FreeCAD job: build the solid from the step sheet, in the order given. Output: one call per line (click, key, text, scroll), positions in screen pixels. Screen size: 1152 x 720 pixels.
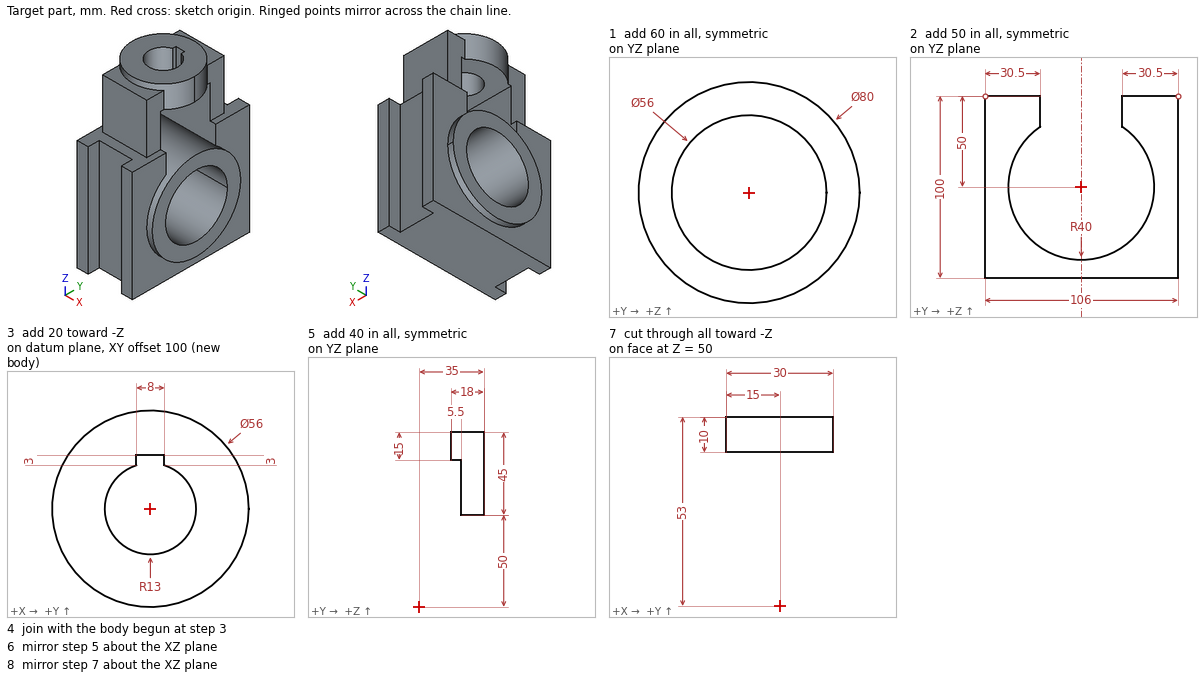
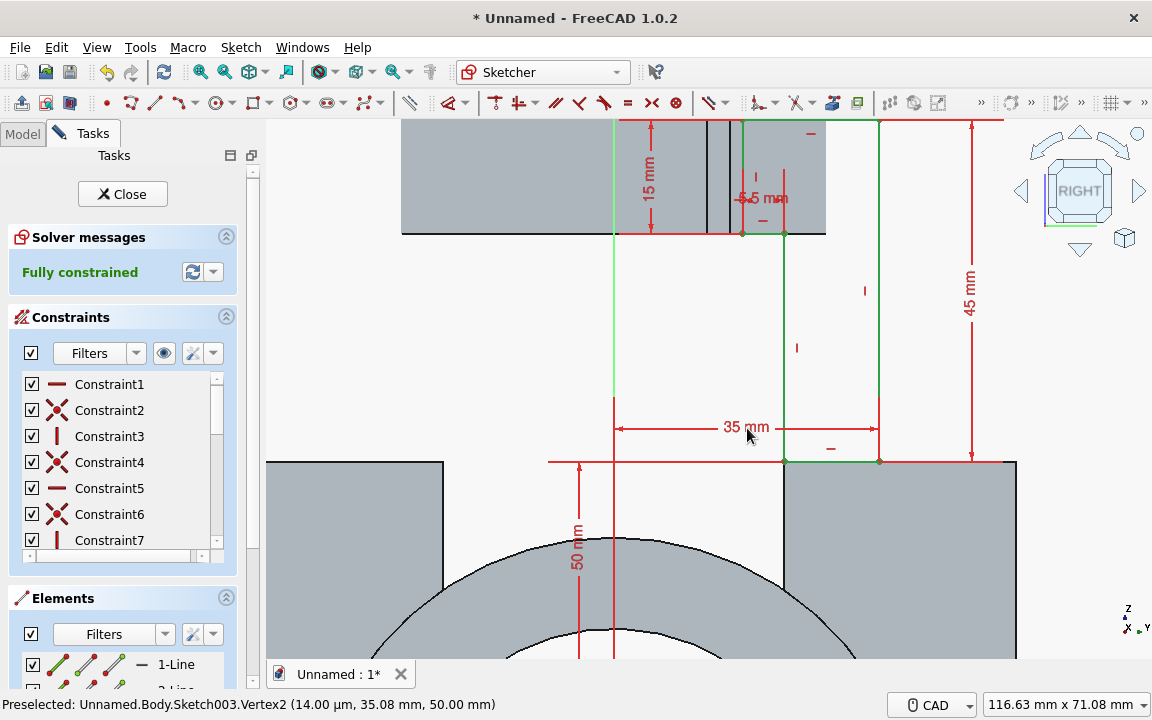
click(123, 194)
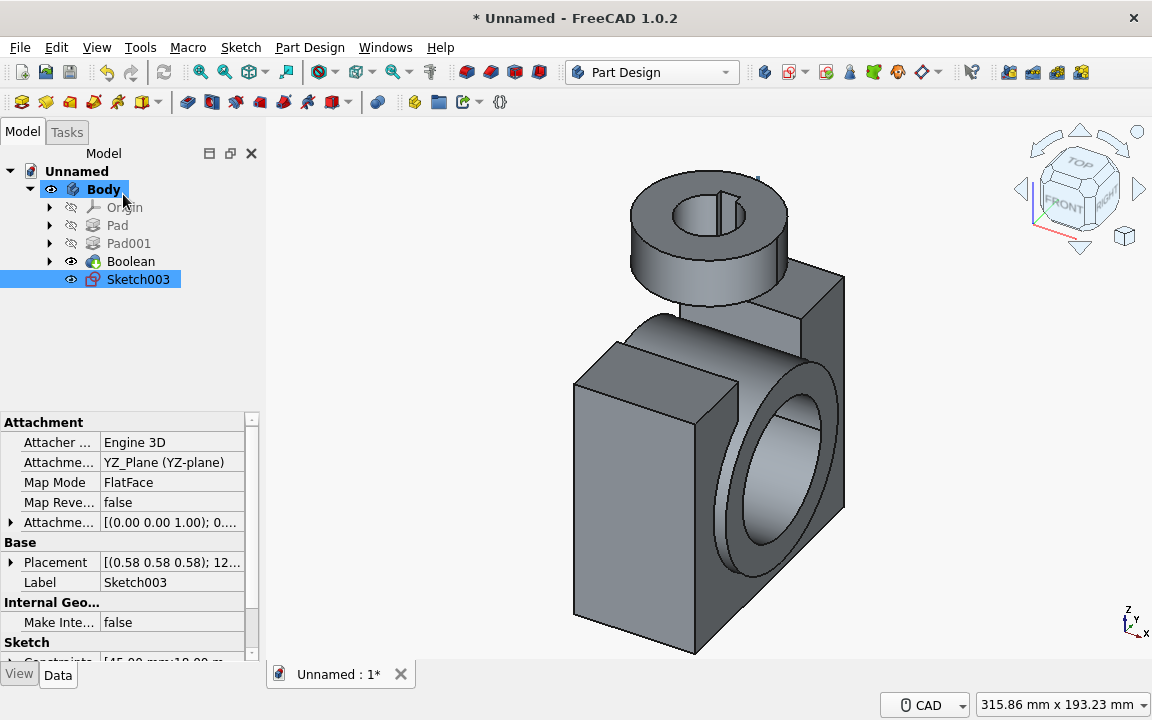
click(22, 102)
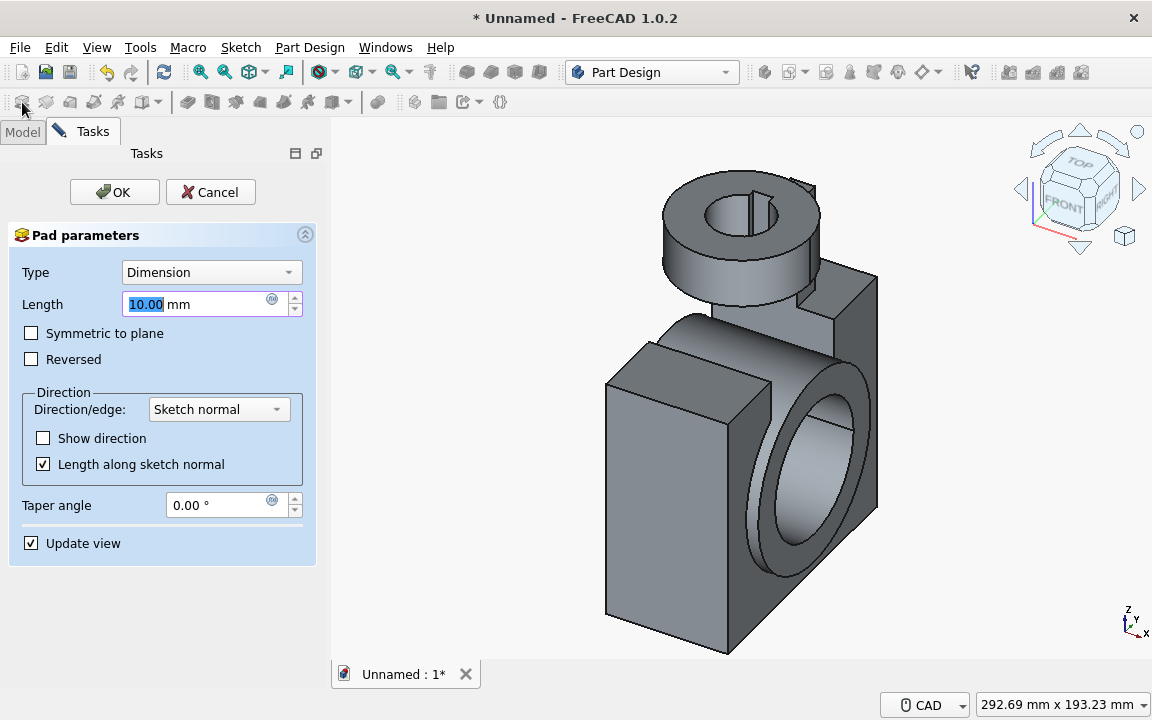
text(40)
key(Tab)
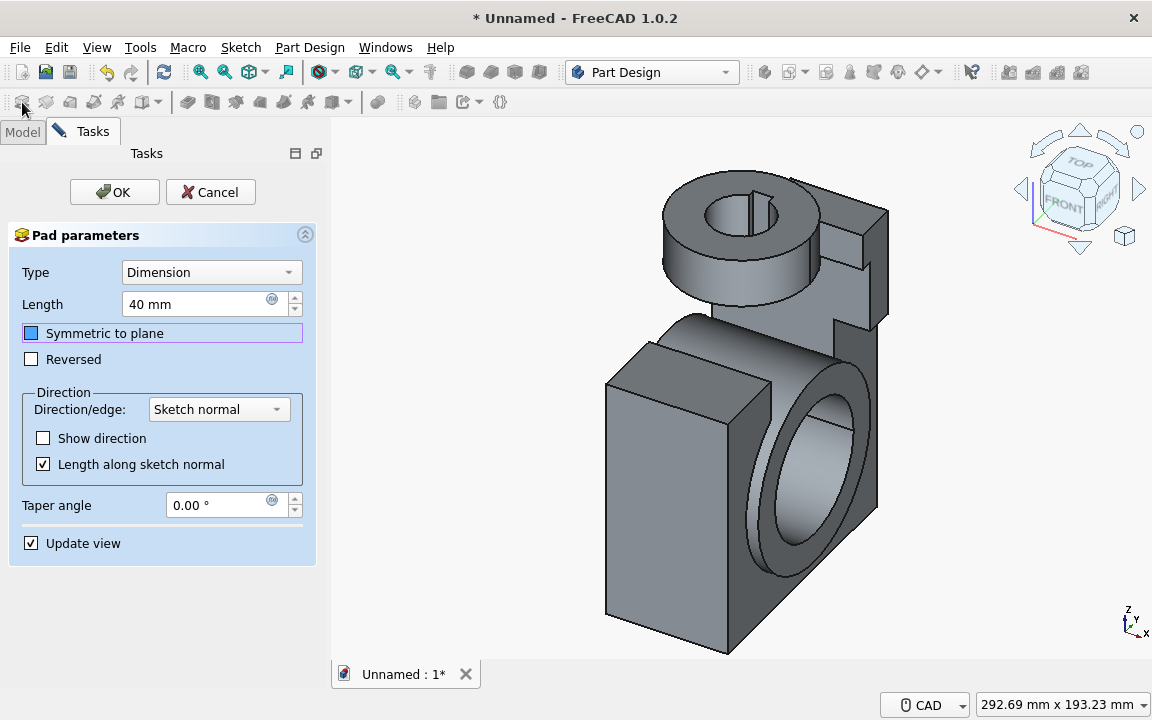
click(30, 333)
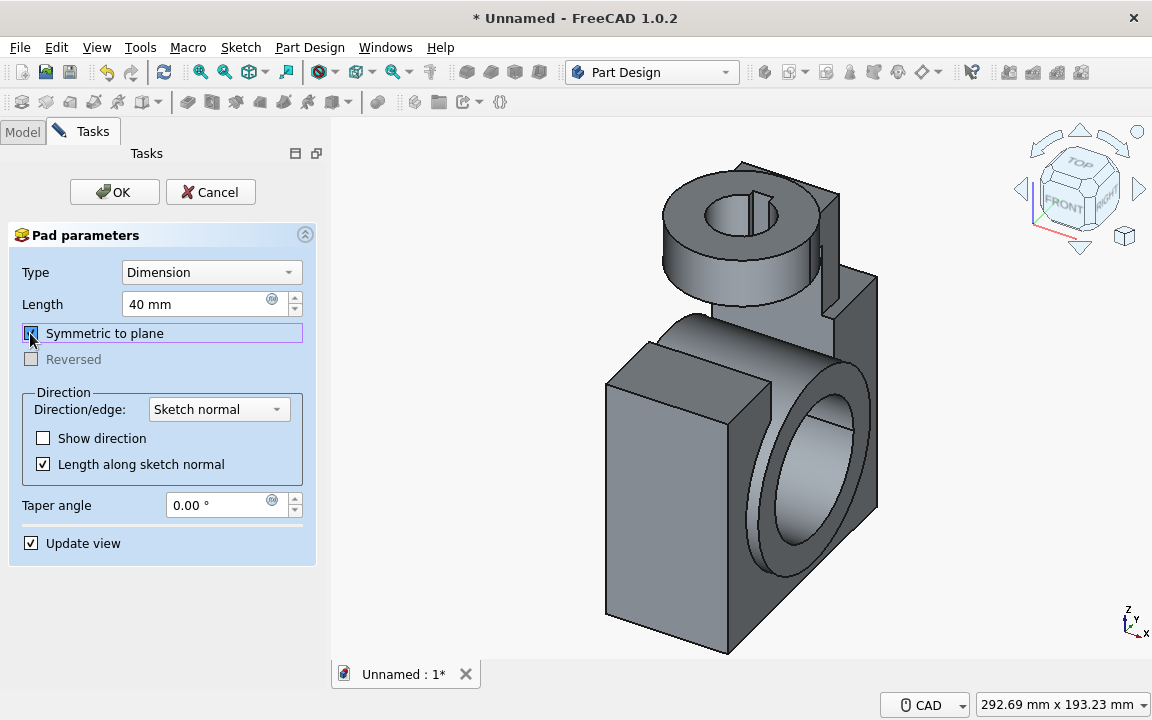
click(115, 192)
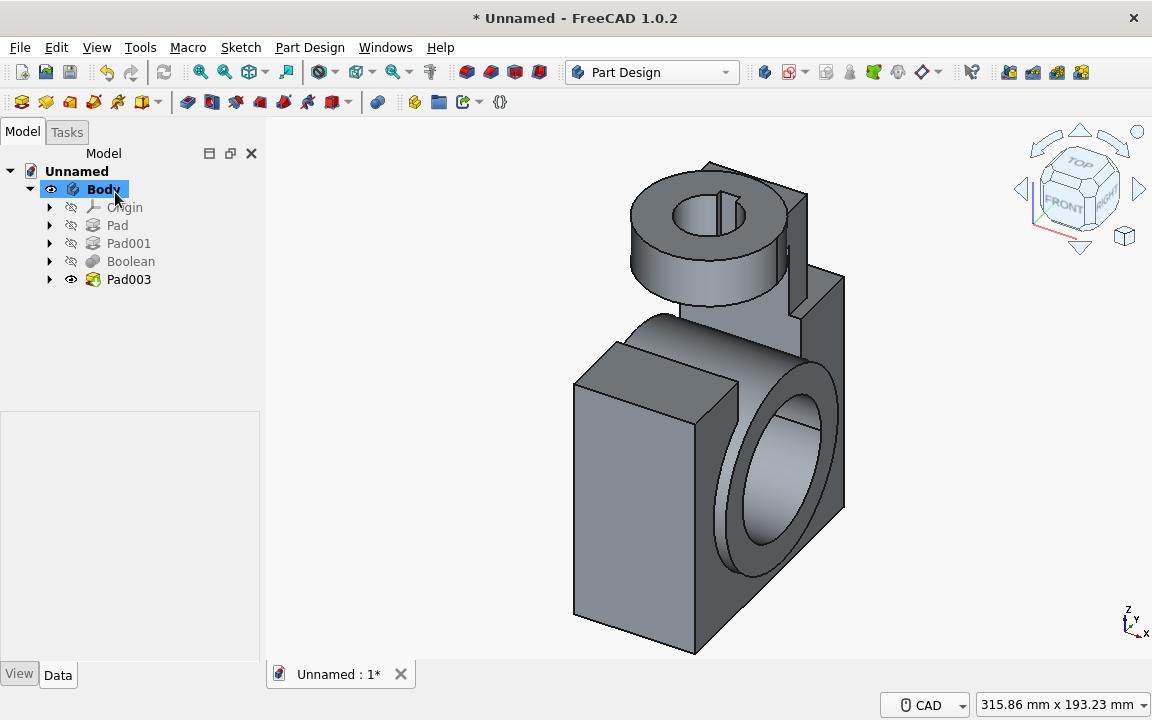
click(116, 279)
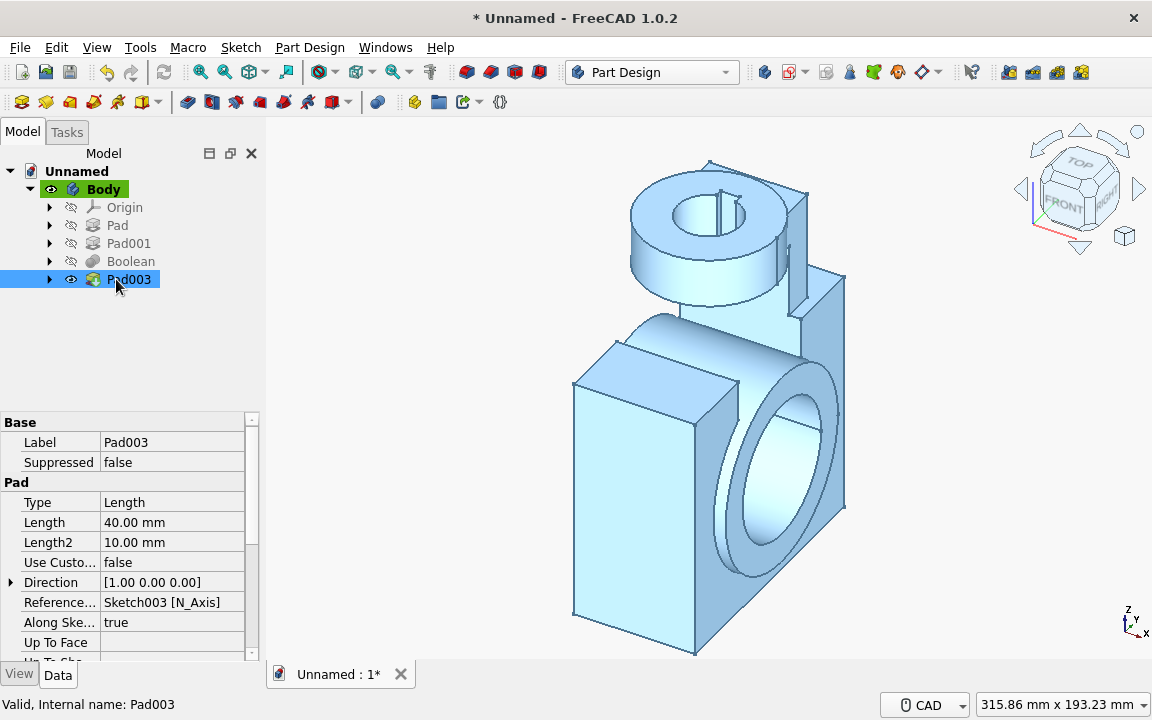
click(1010, 72)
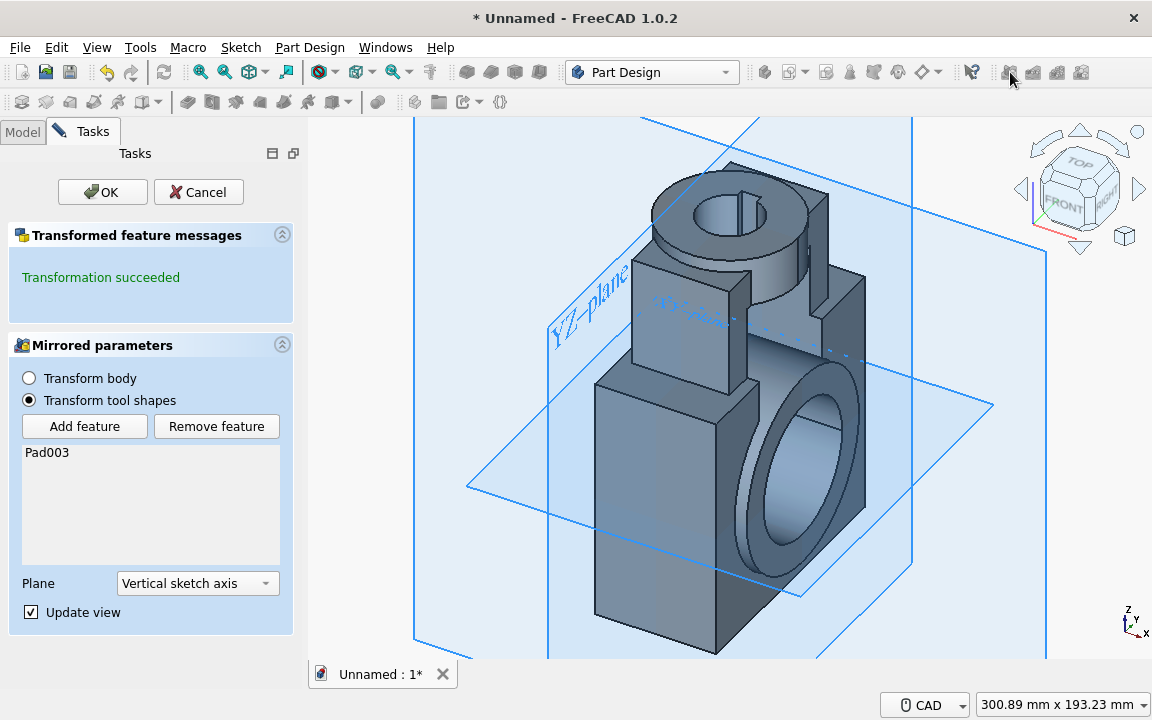
click(198, 584)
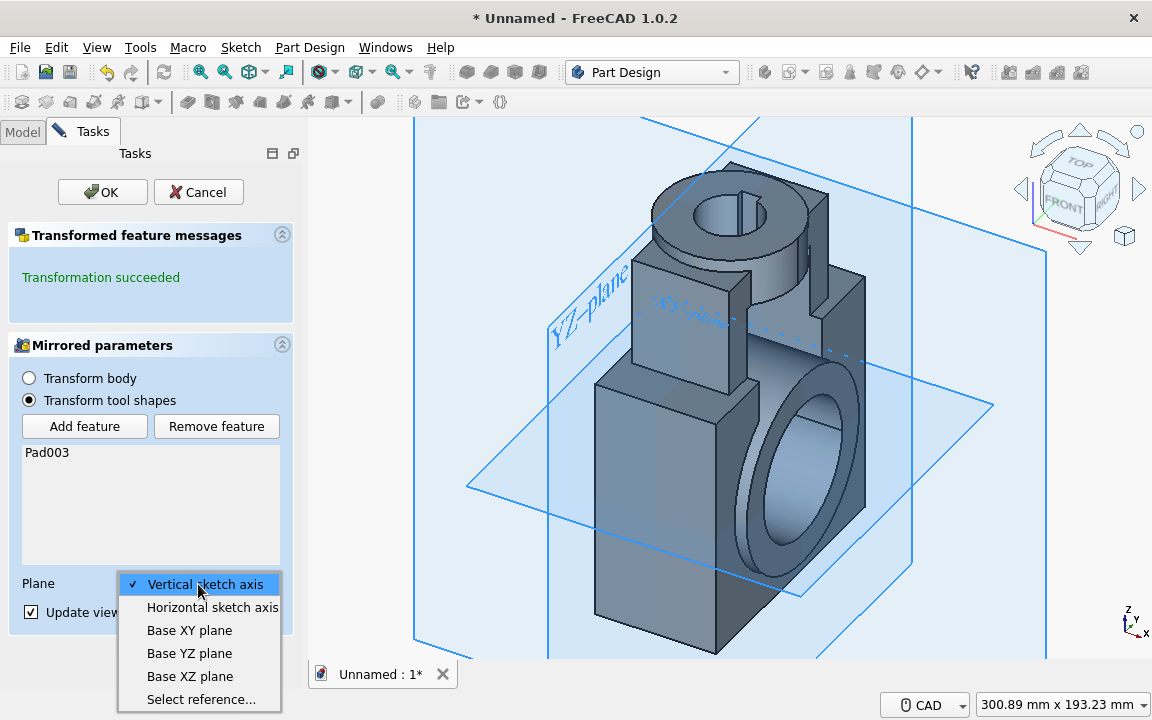
click(198, 676)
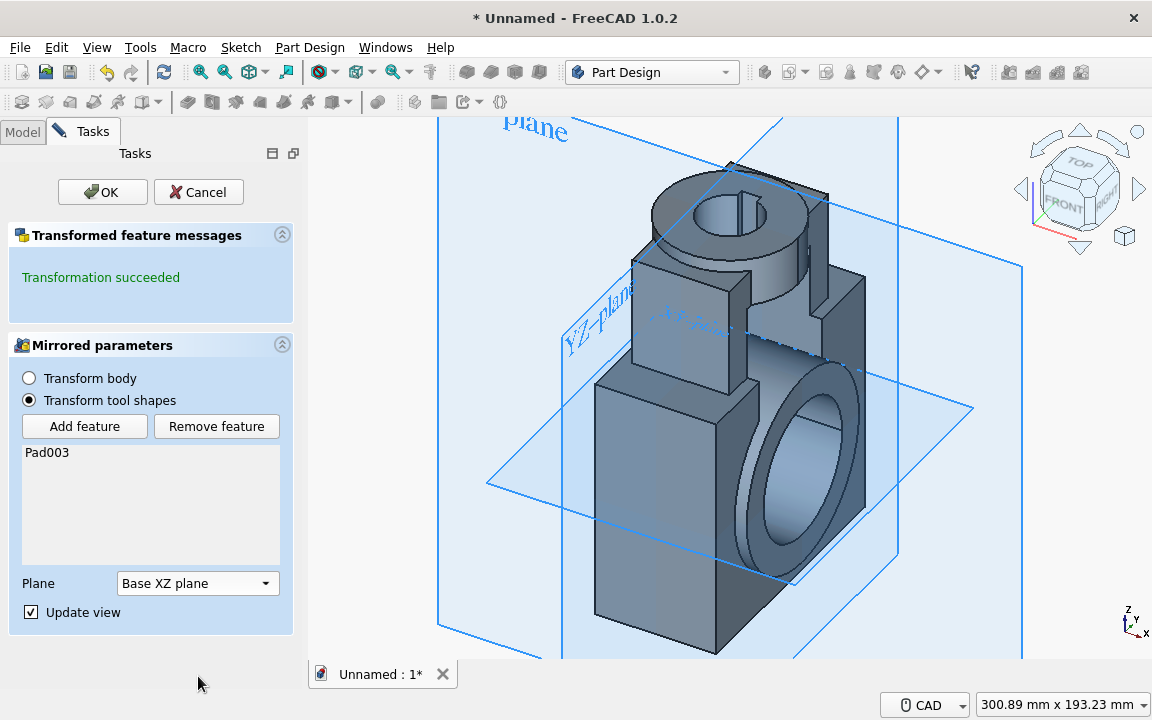
click(103, 192)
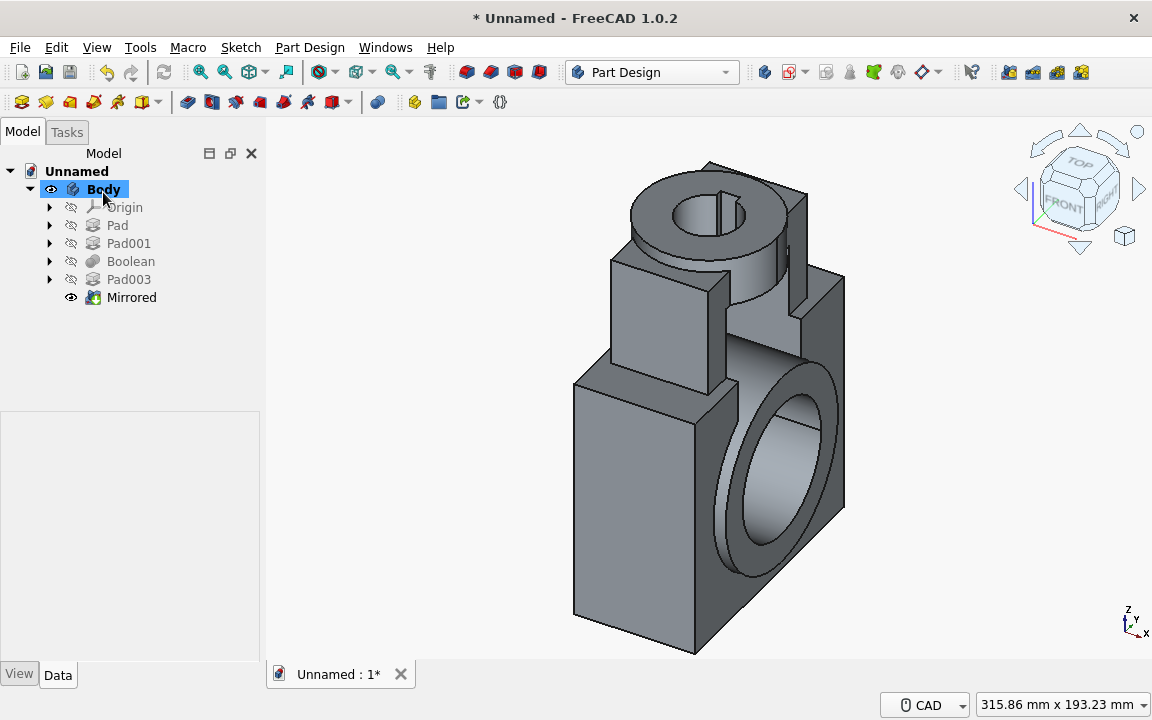
key(0)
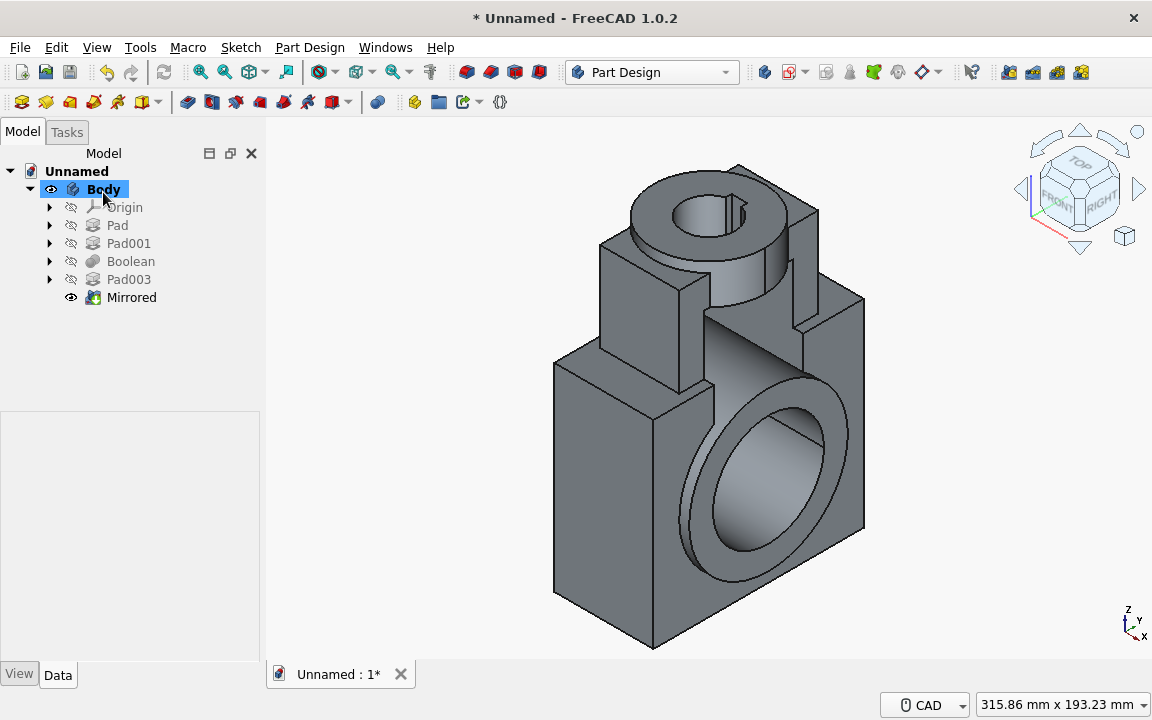
click(829, 293)